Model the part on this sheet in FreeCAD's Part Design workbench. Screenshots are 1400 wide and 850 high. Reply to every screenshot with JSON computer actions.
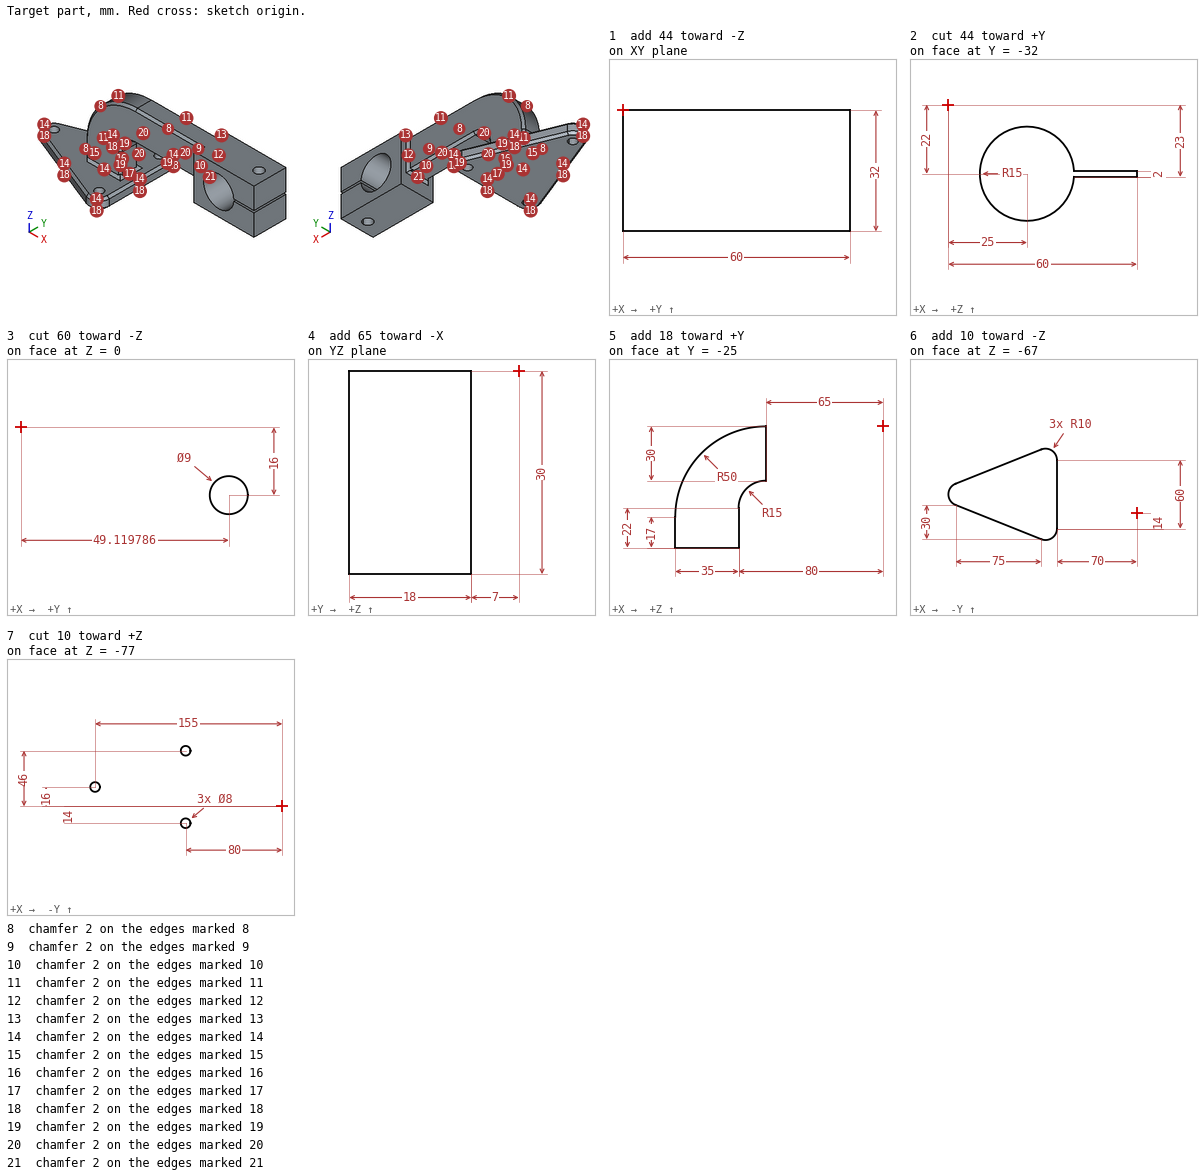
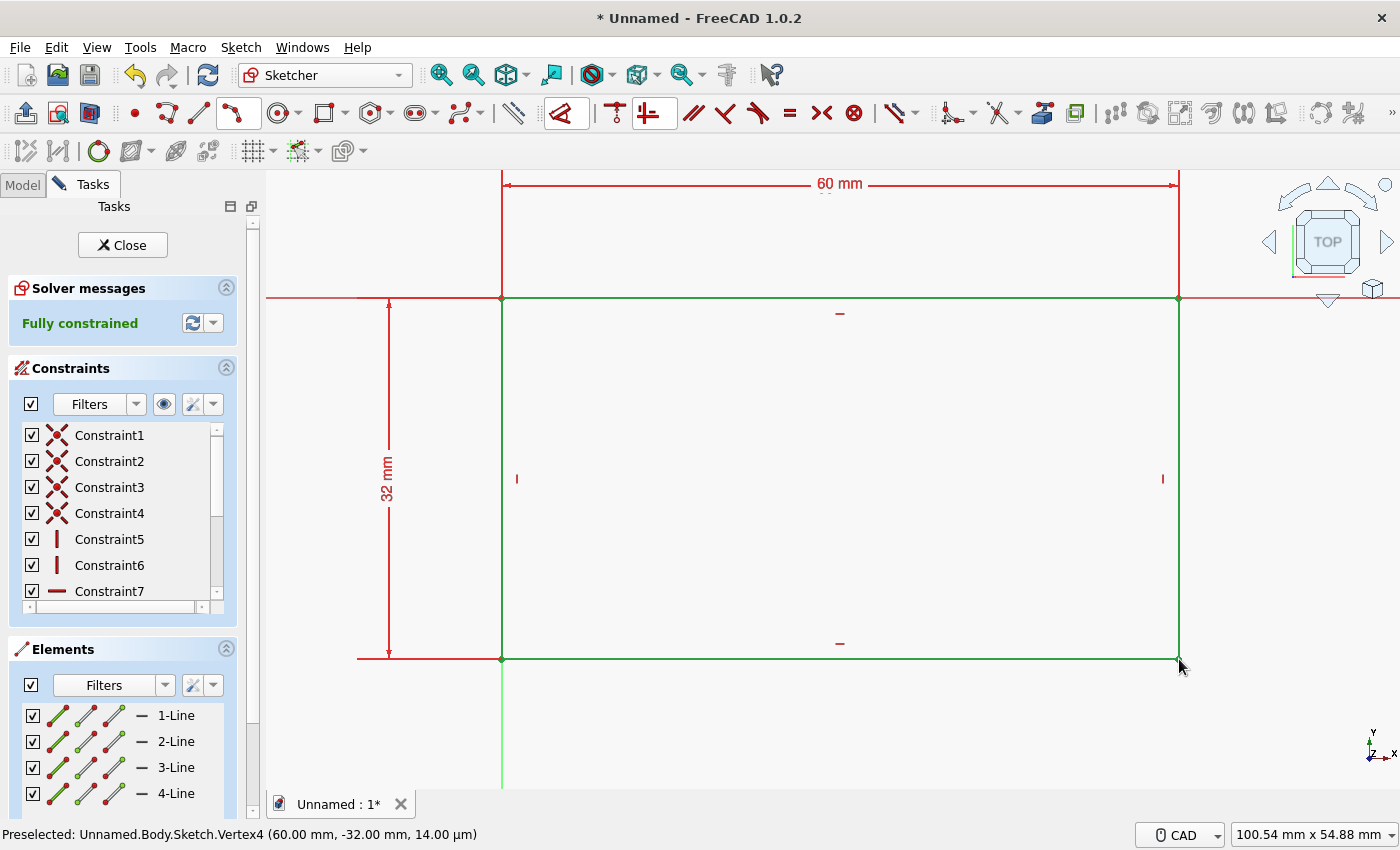
{"action": "left_click", "coordinate": [123, 245]}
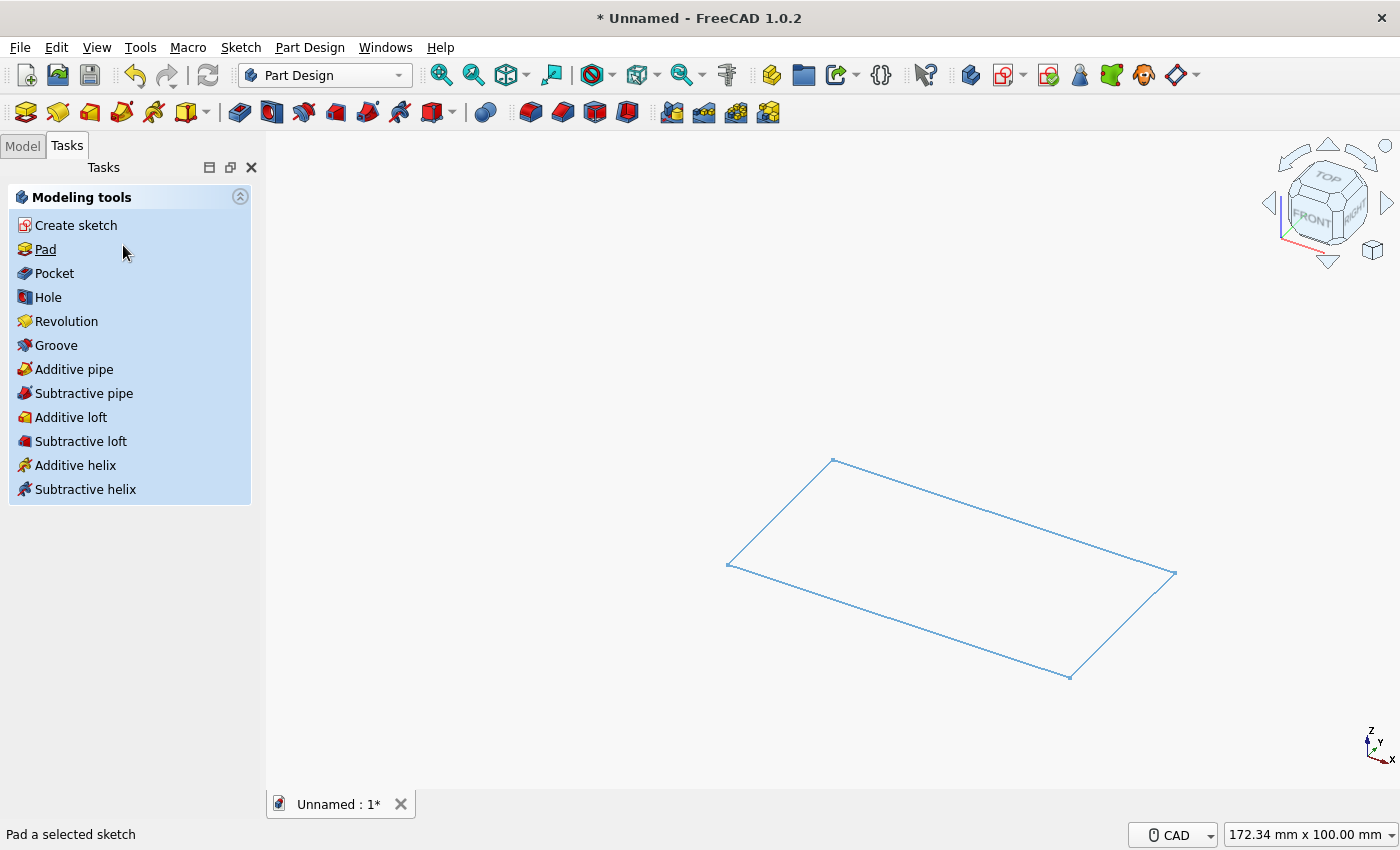
{"action": "left_click", "coordinate": [26, 112]}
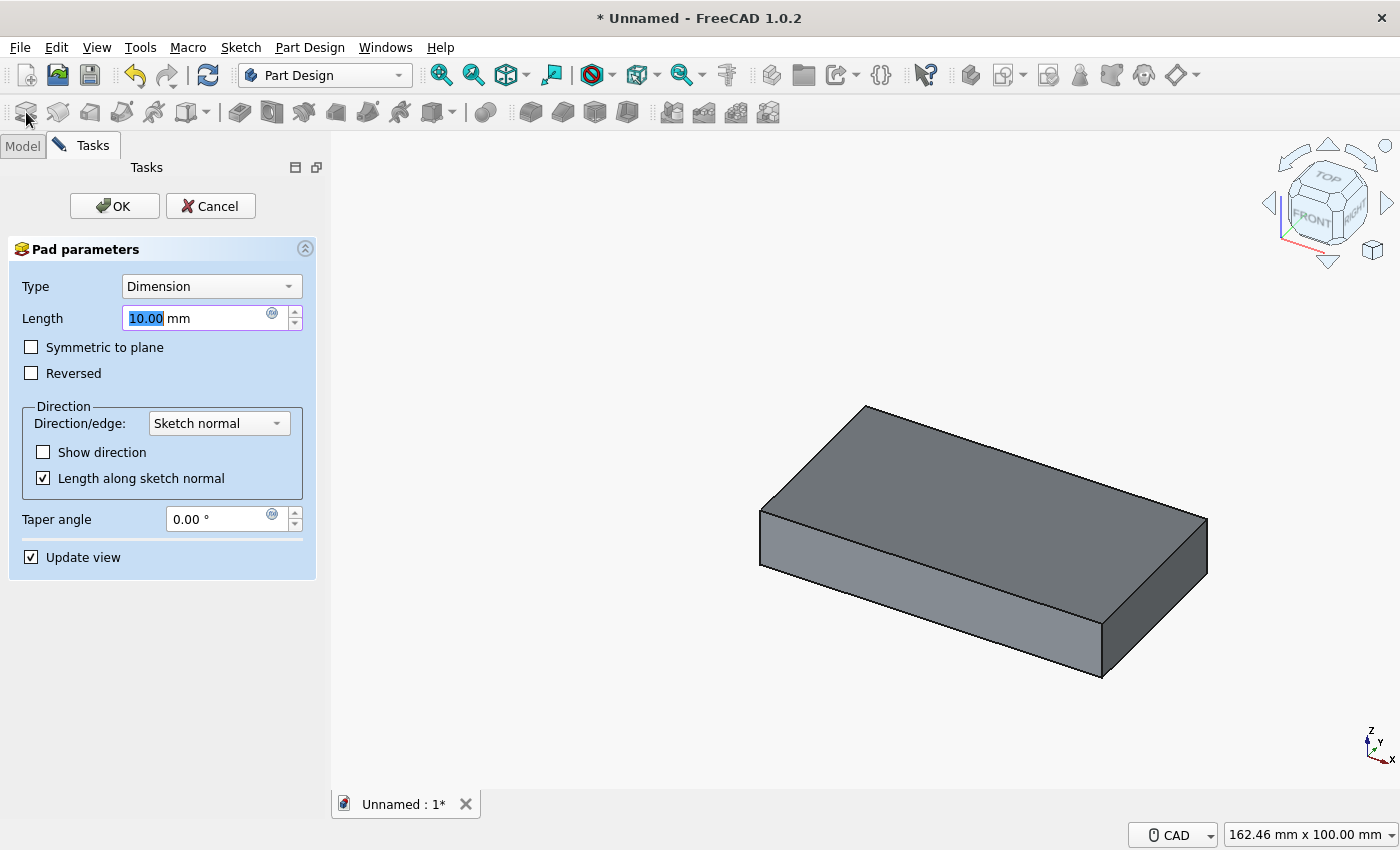
{"action": "type", "text": "44"}
{"action": "key", "text": "Tab"}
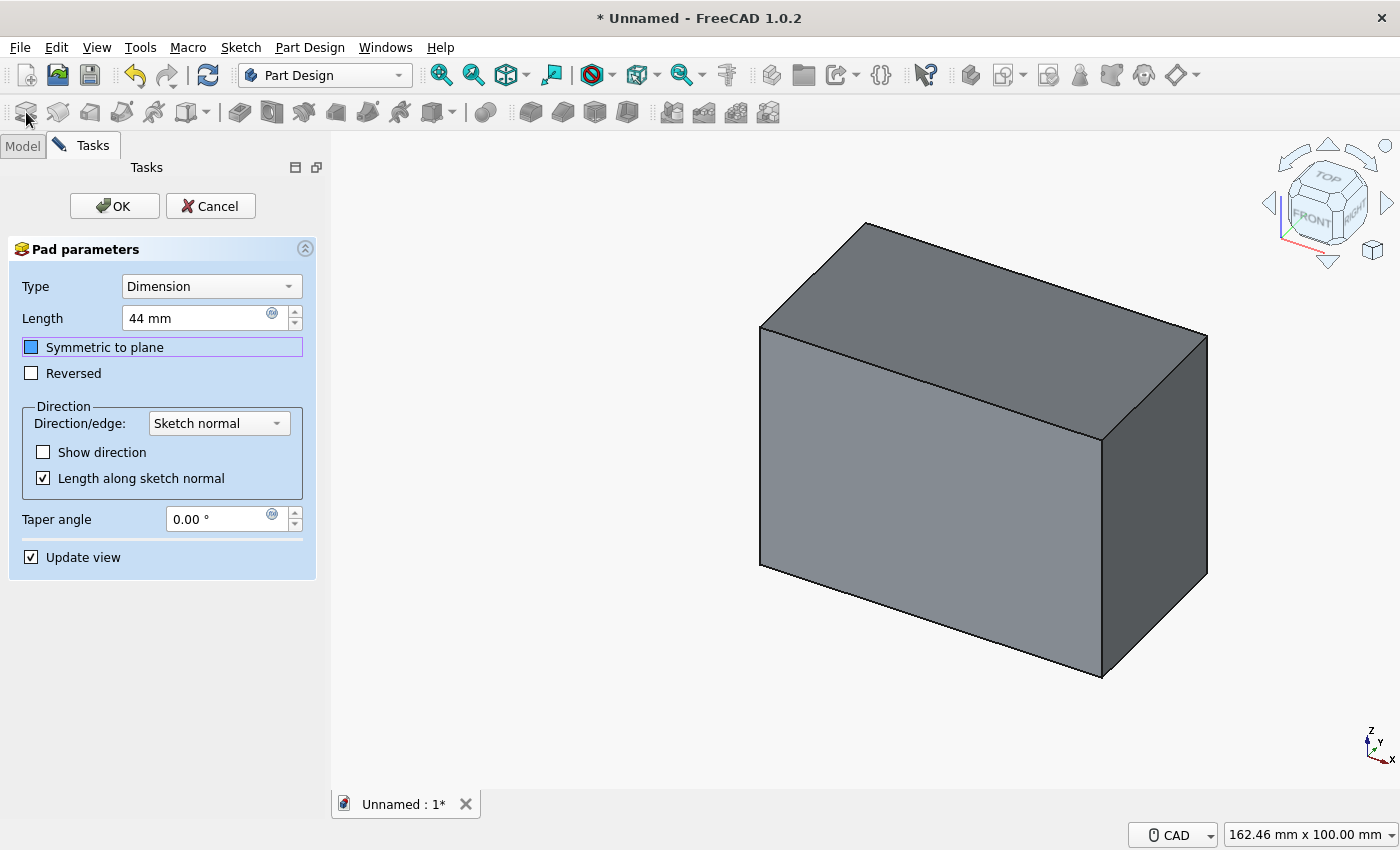
{"action": "left_click", "coordinate": [30, 373]}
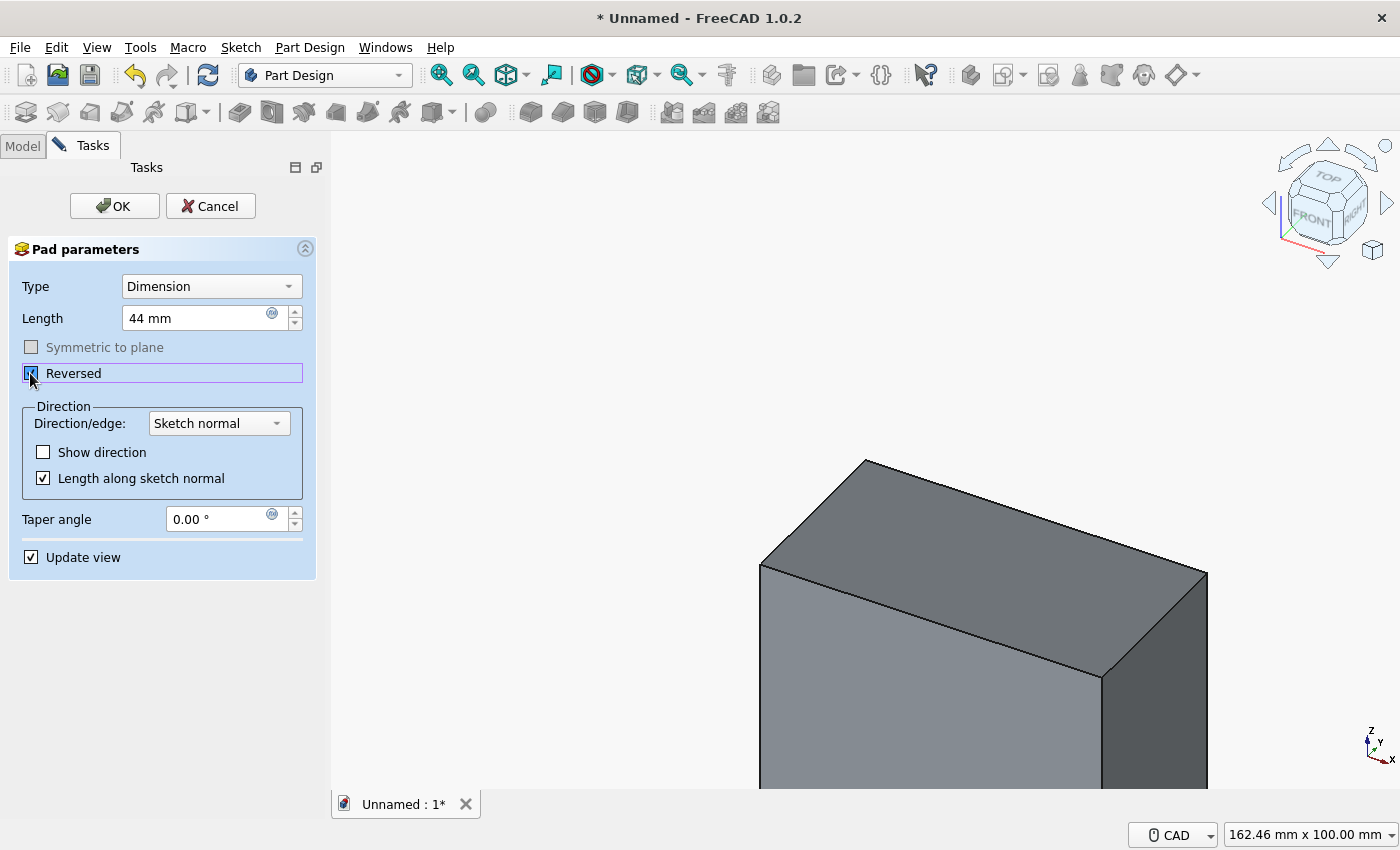
{"action": "left_click", "coordinate": [115, 206]}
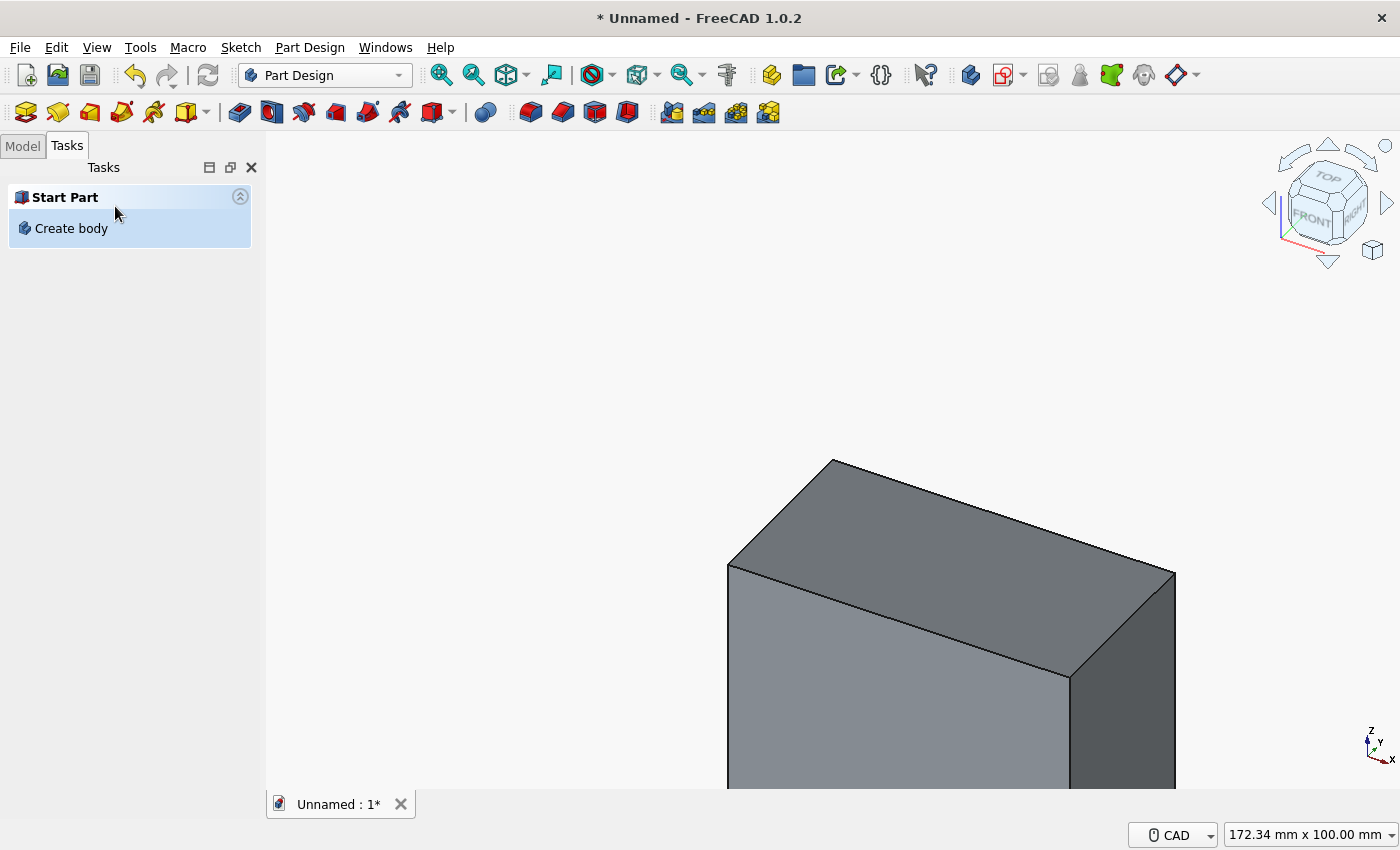
{"action": "left_click", "coordinate": [442, 76]}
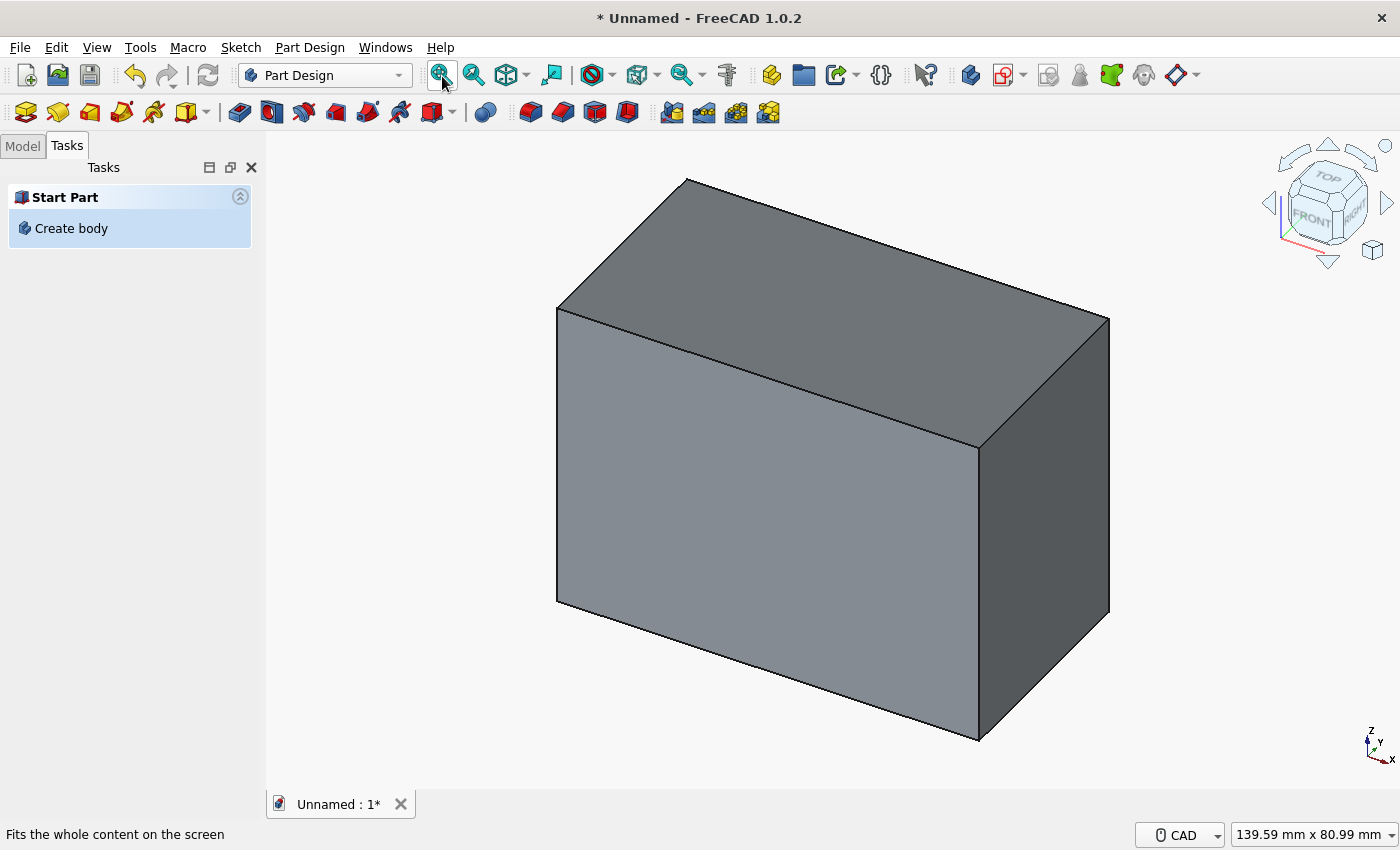
{"action": "left_click", "coordinate": [768, 524]}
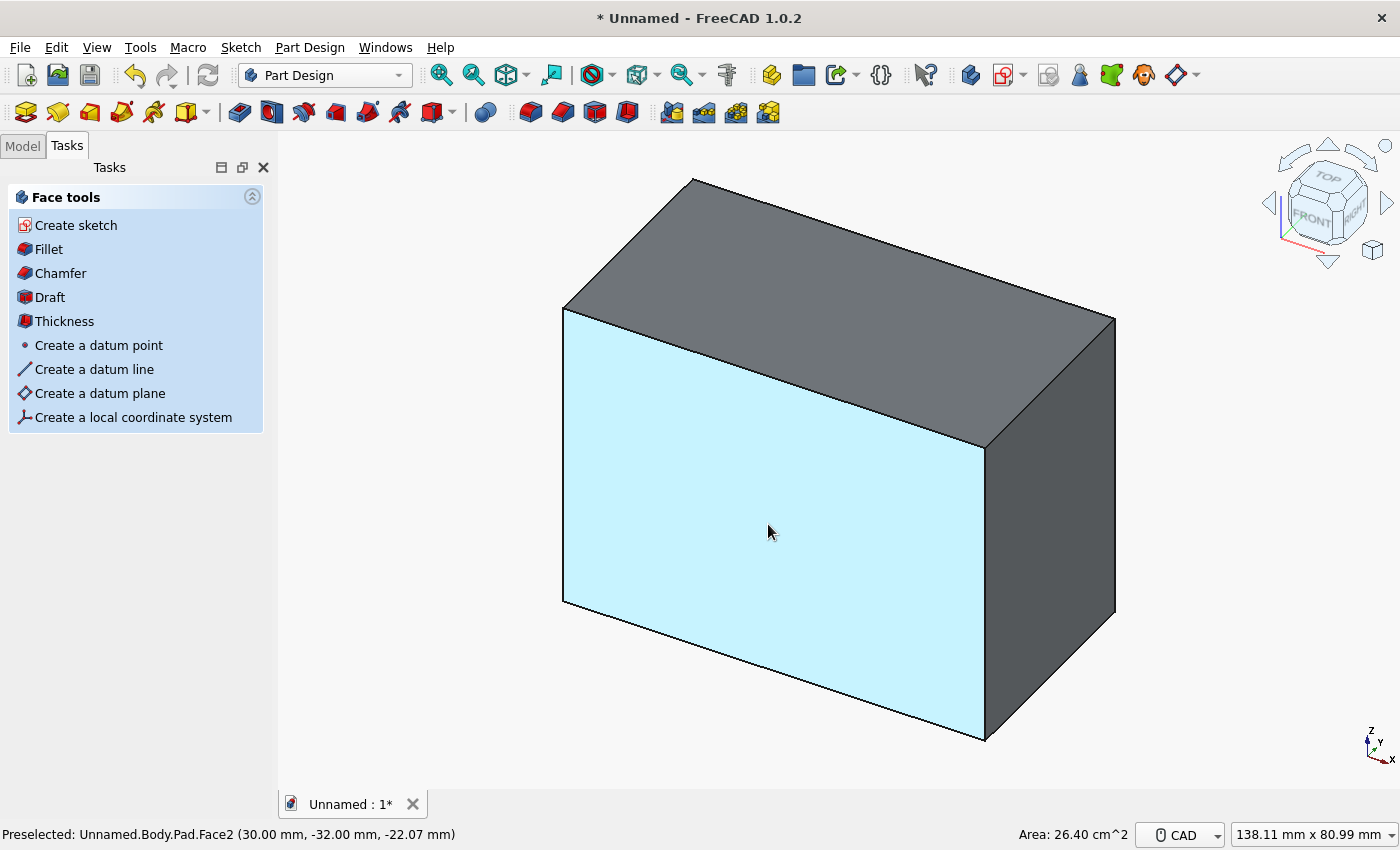
{"action": "left_click", "coordinate": [1004, 76]}